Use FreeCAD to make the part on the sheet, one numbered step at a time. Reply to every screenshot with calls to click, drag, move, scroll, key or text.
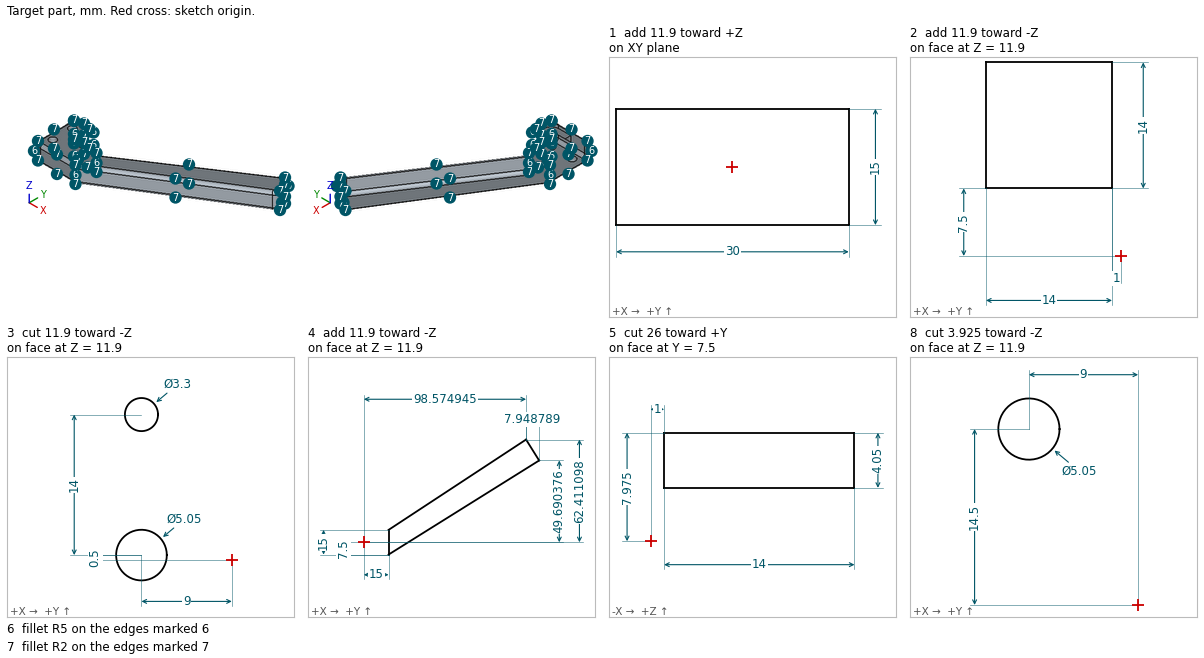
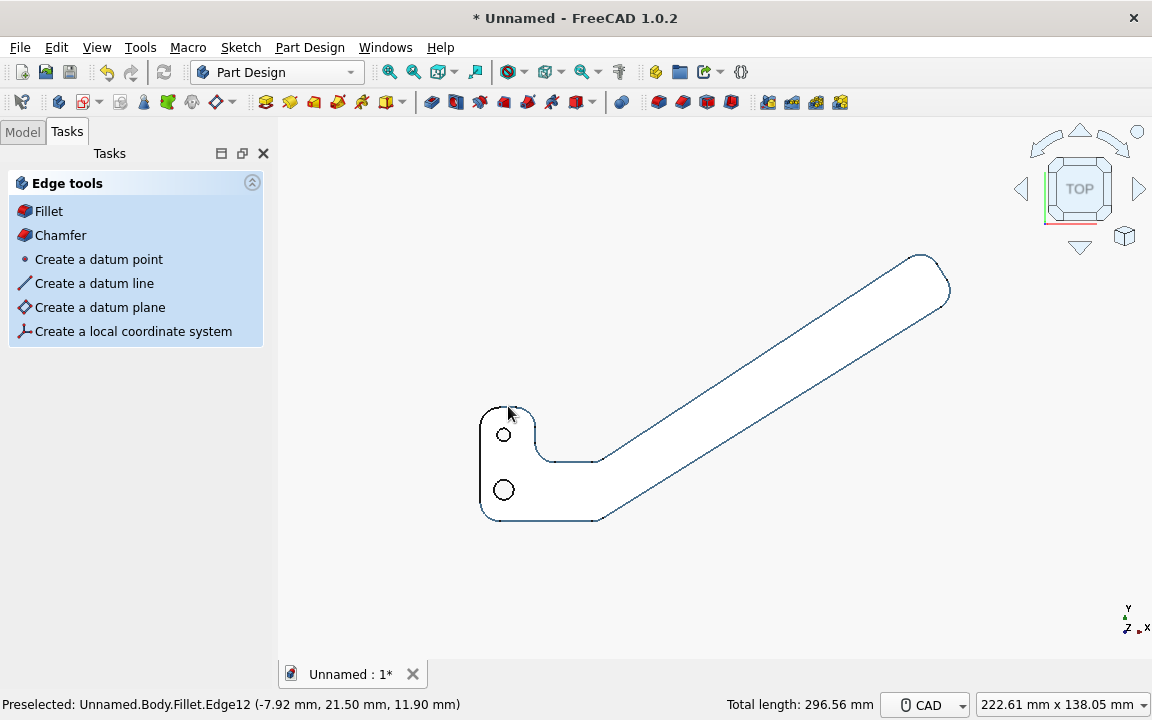
click(480, 463, ctrl)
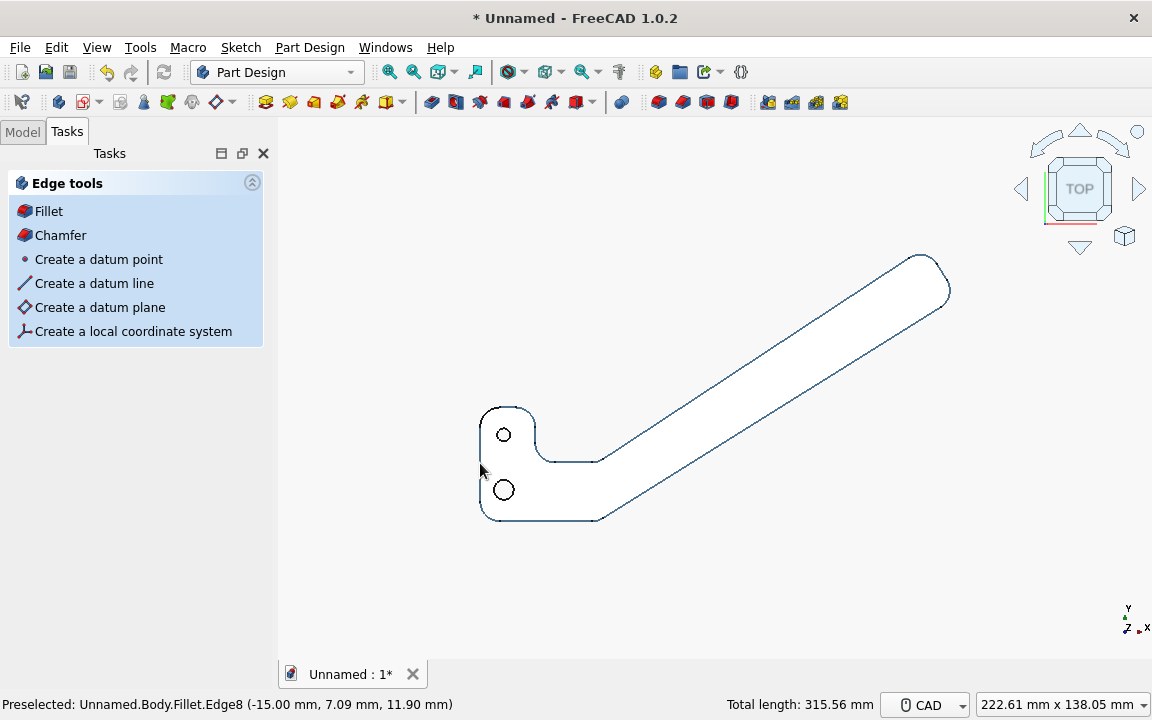
click(486, 412, ctrl)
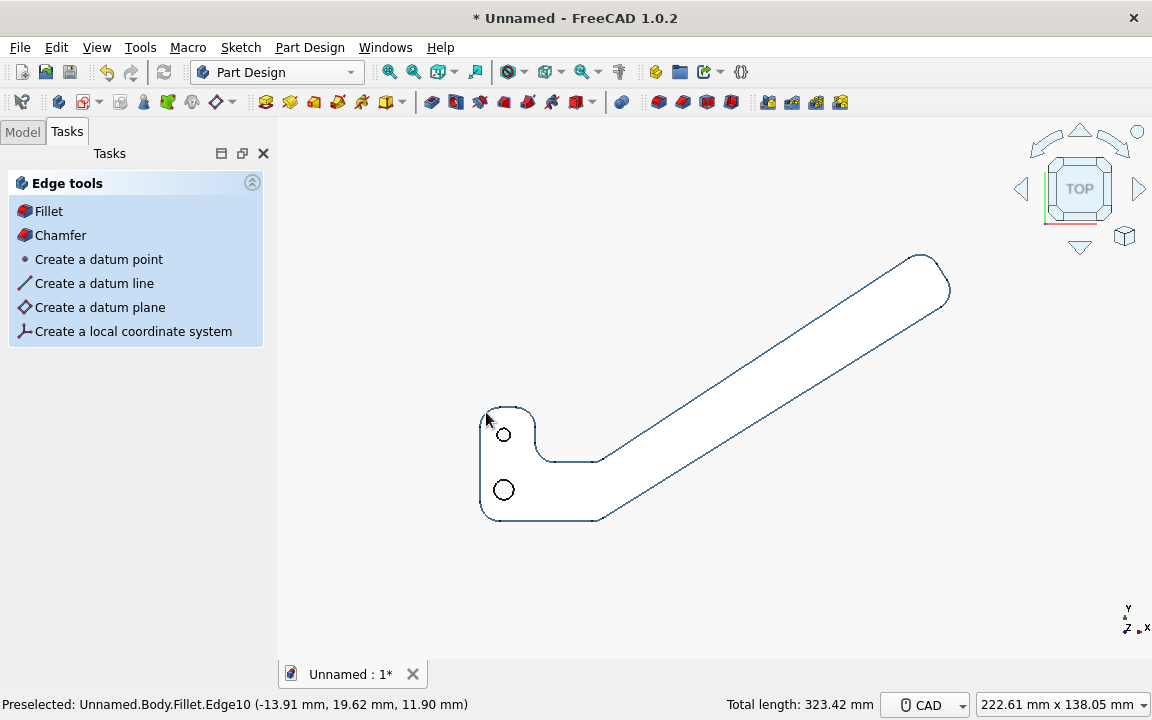
scroll(598, 461, up, 7)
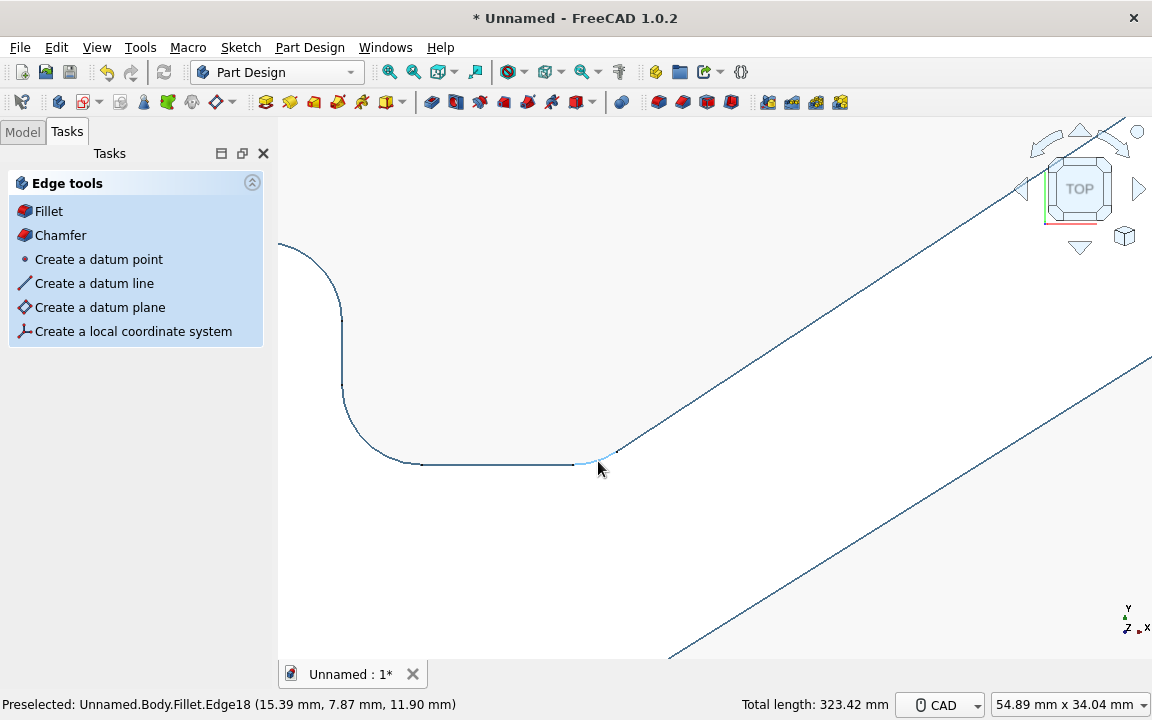
click(390, 72)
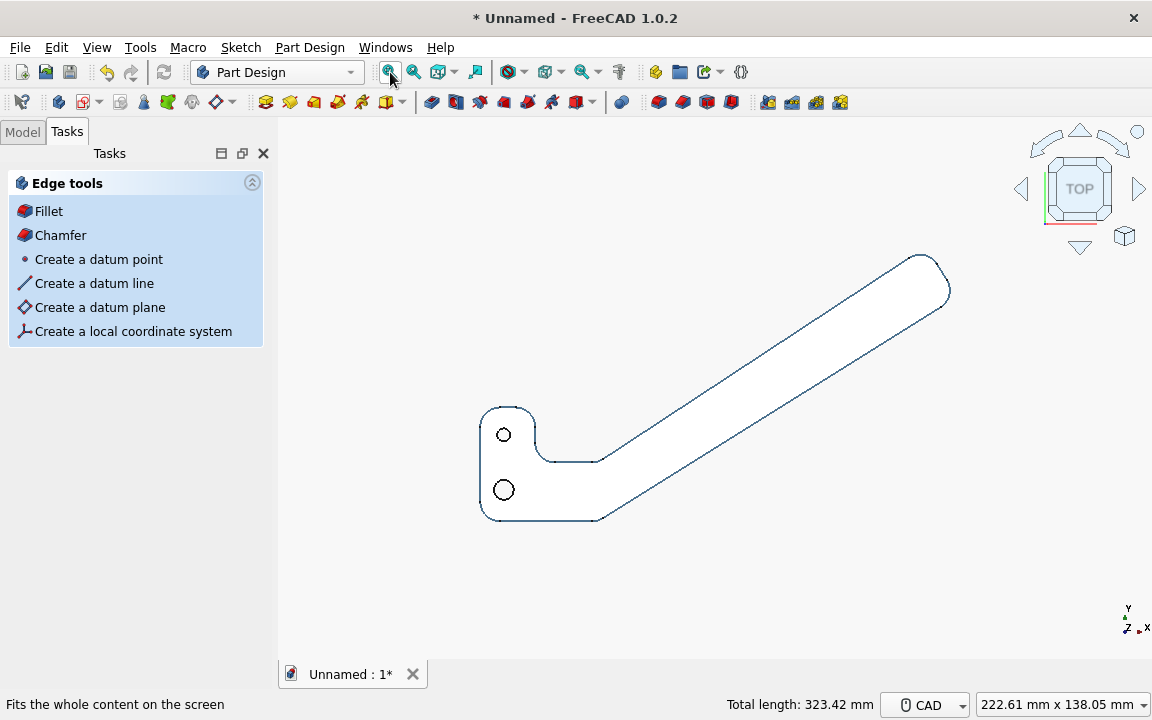
key(0)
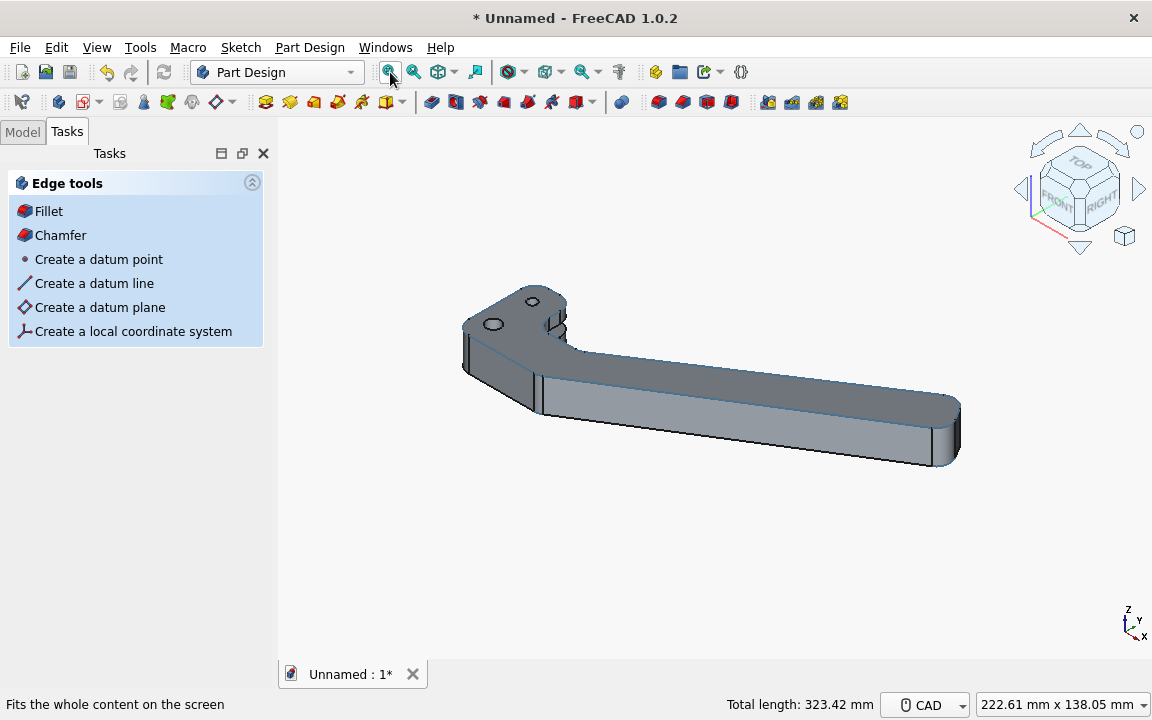
scroll(580, 388, up, 7)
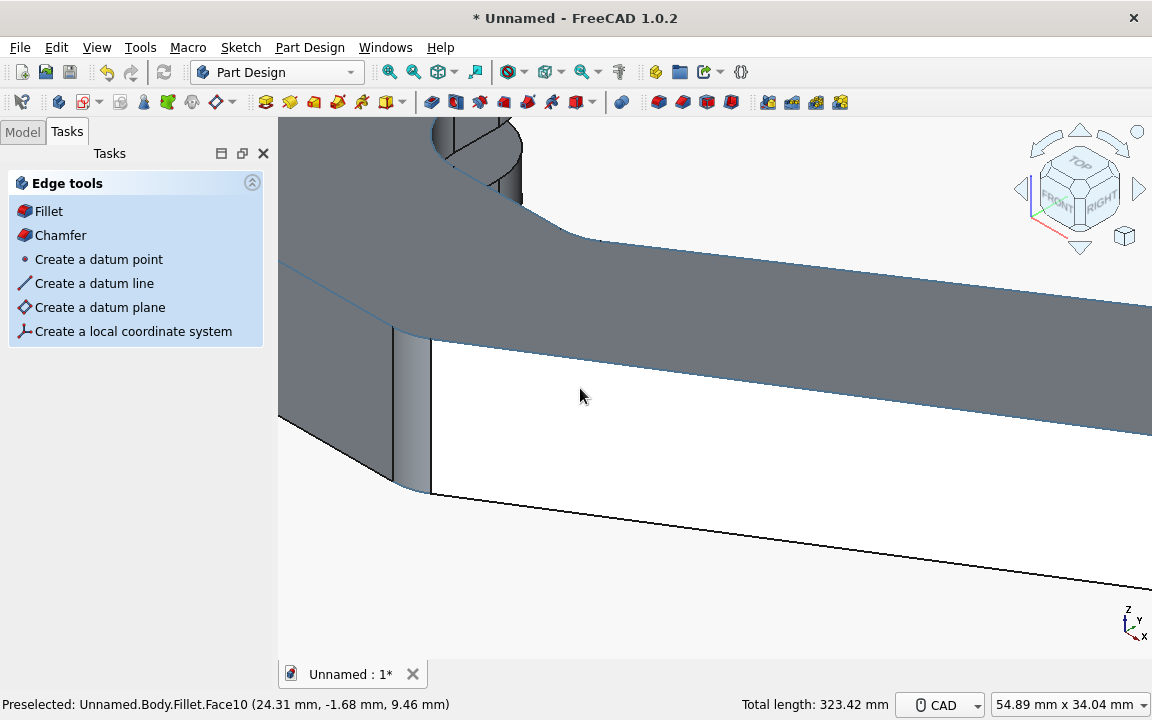
click(390, 72)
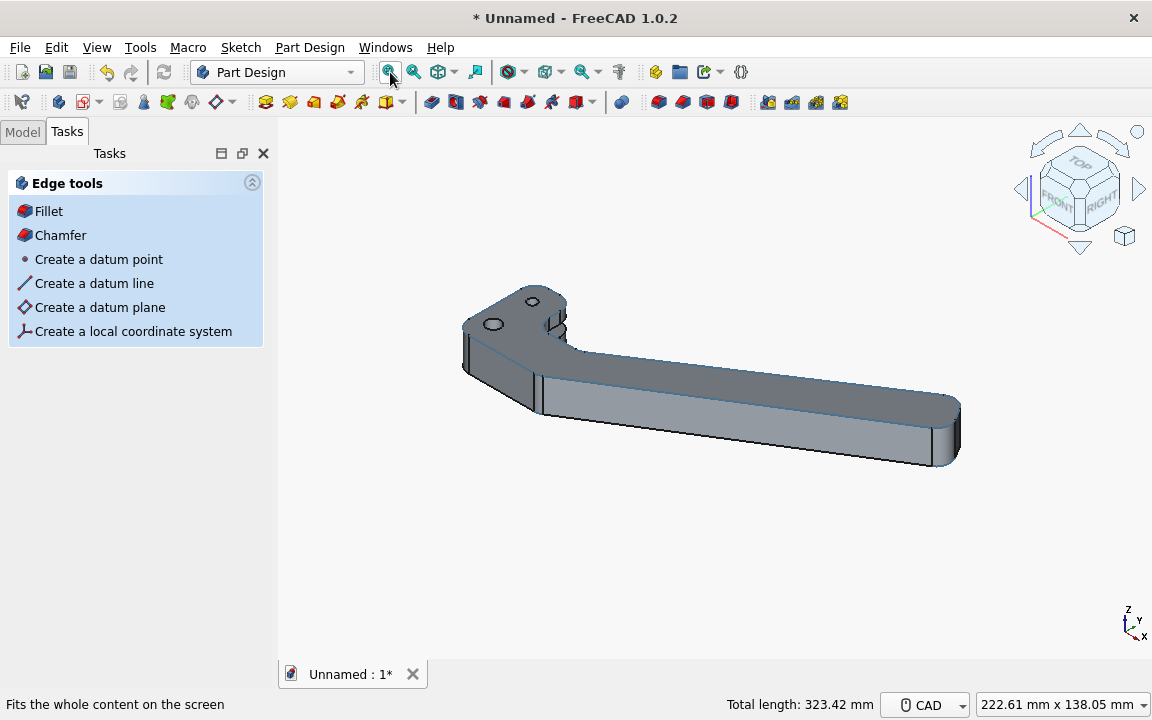
key(1)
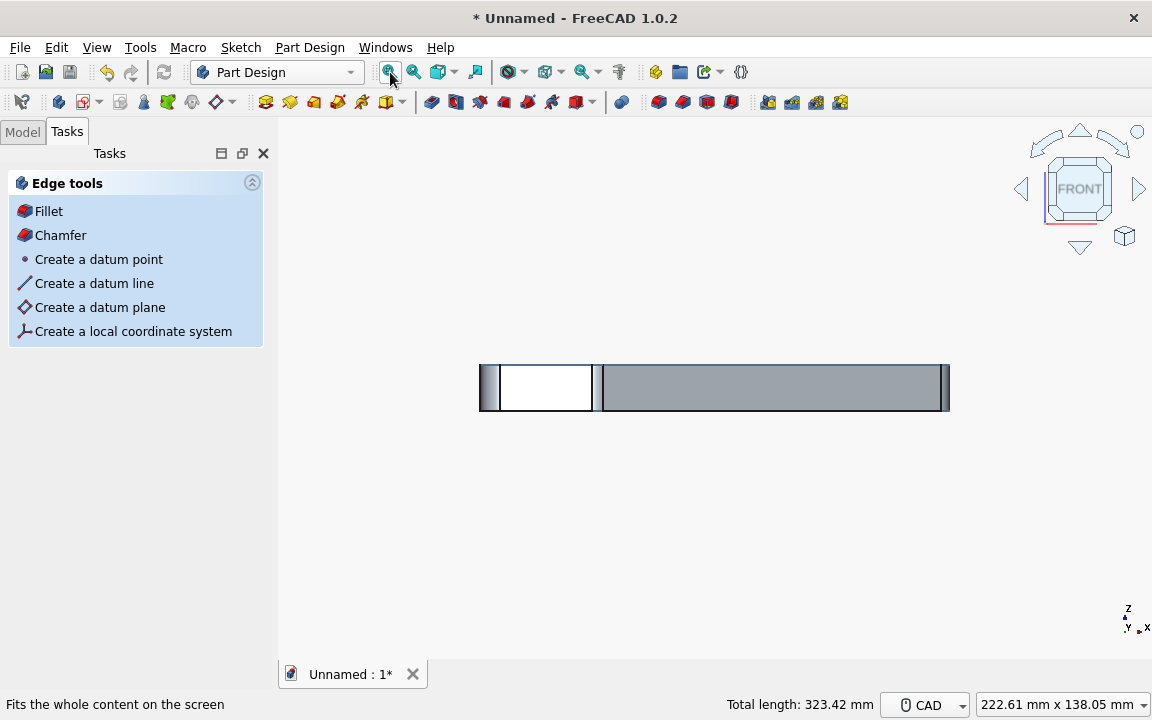
click(772, 410, ctrl)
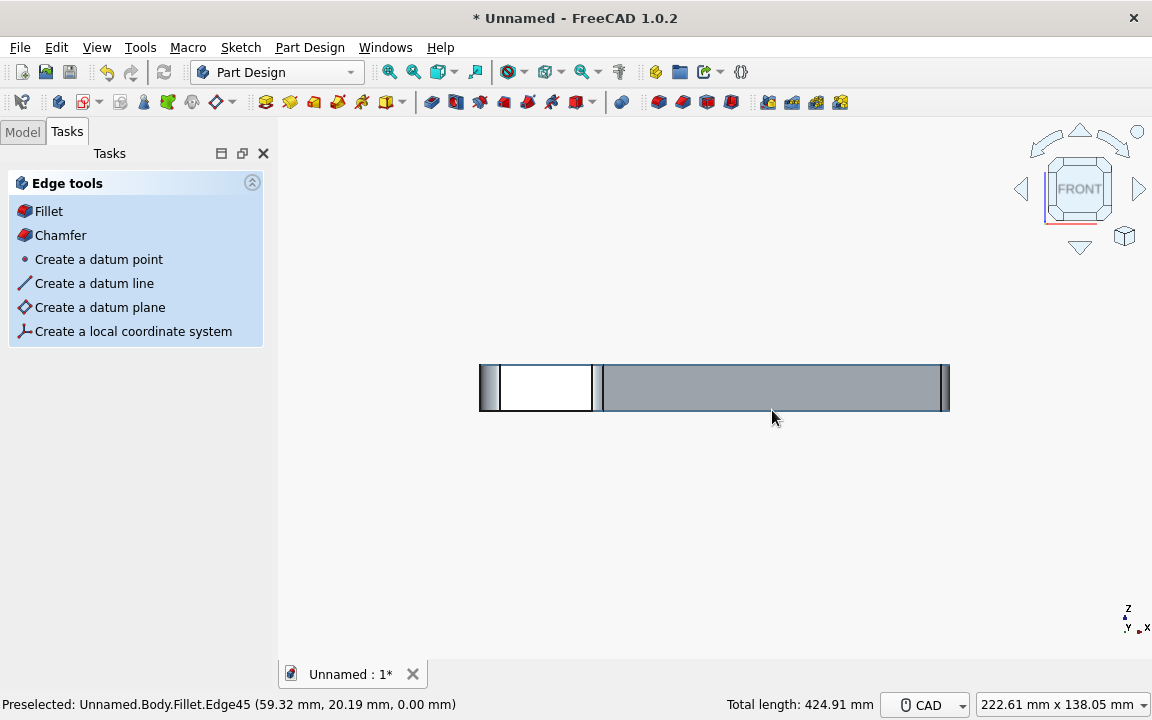
click(546, 410, ctrl)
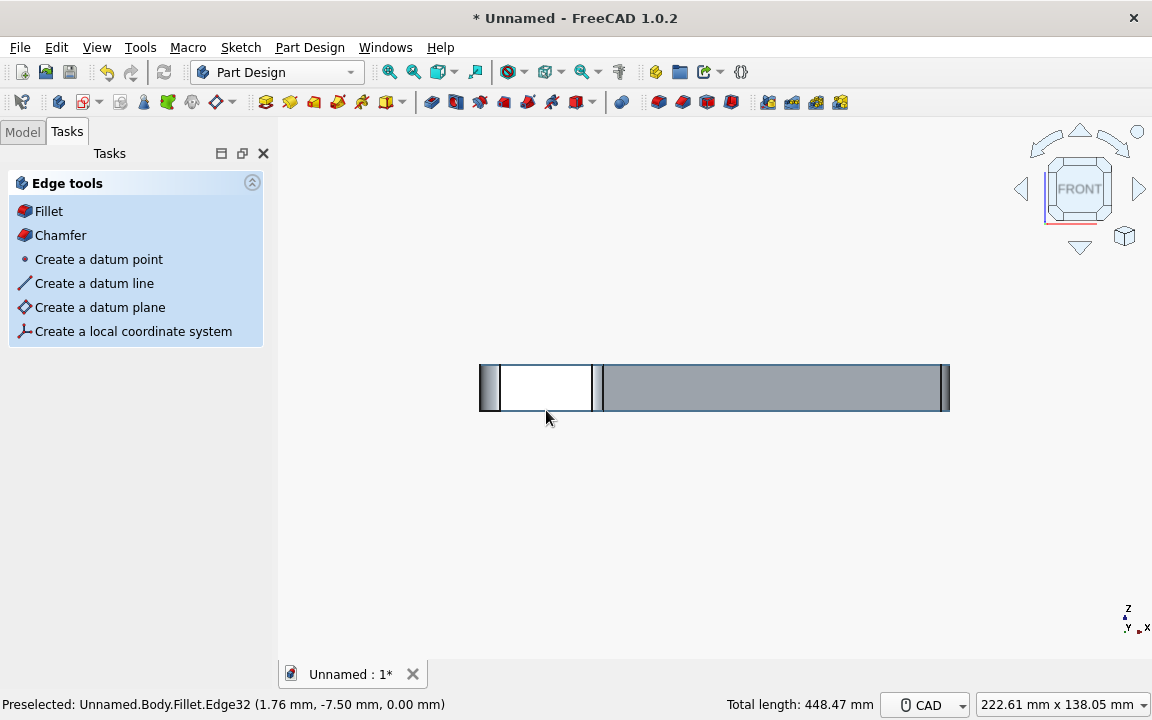
click(486, 410, ctrl)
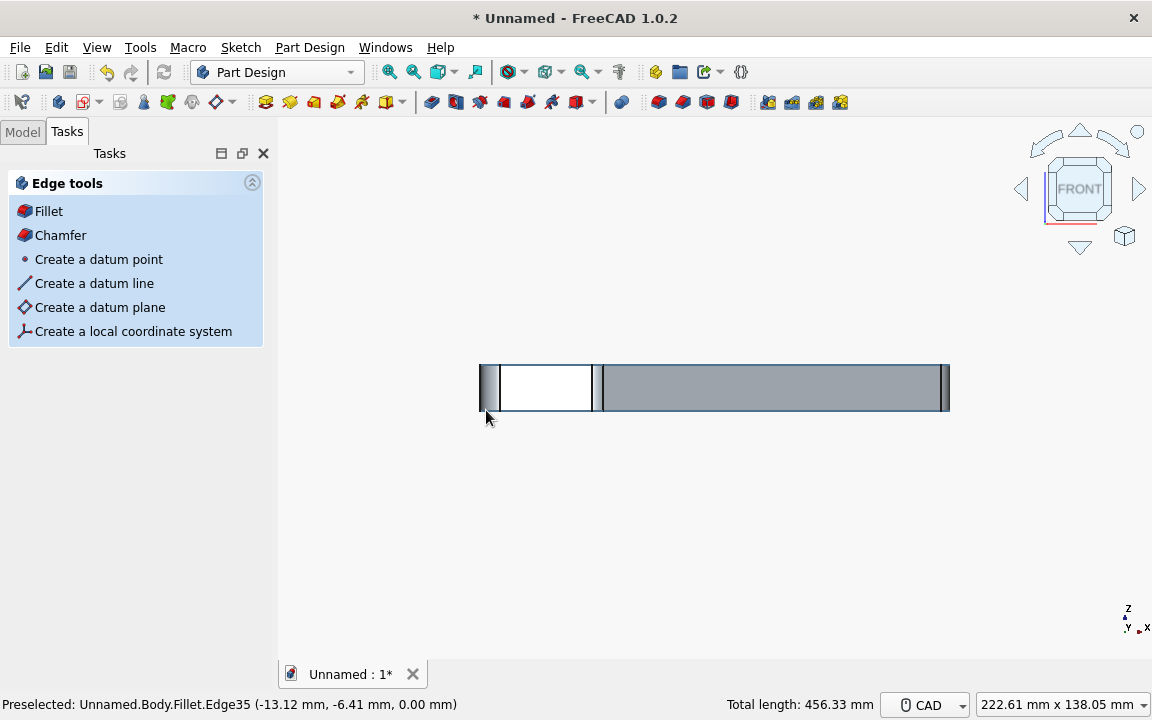
scroll(598, 410, up, 7)